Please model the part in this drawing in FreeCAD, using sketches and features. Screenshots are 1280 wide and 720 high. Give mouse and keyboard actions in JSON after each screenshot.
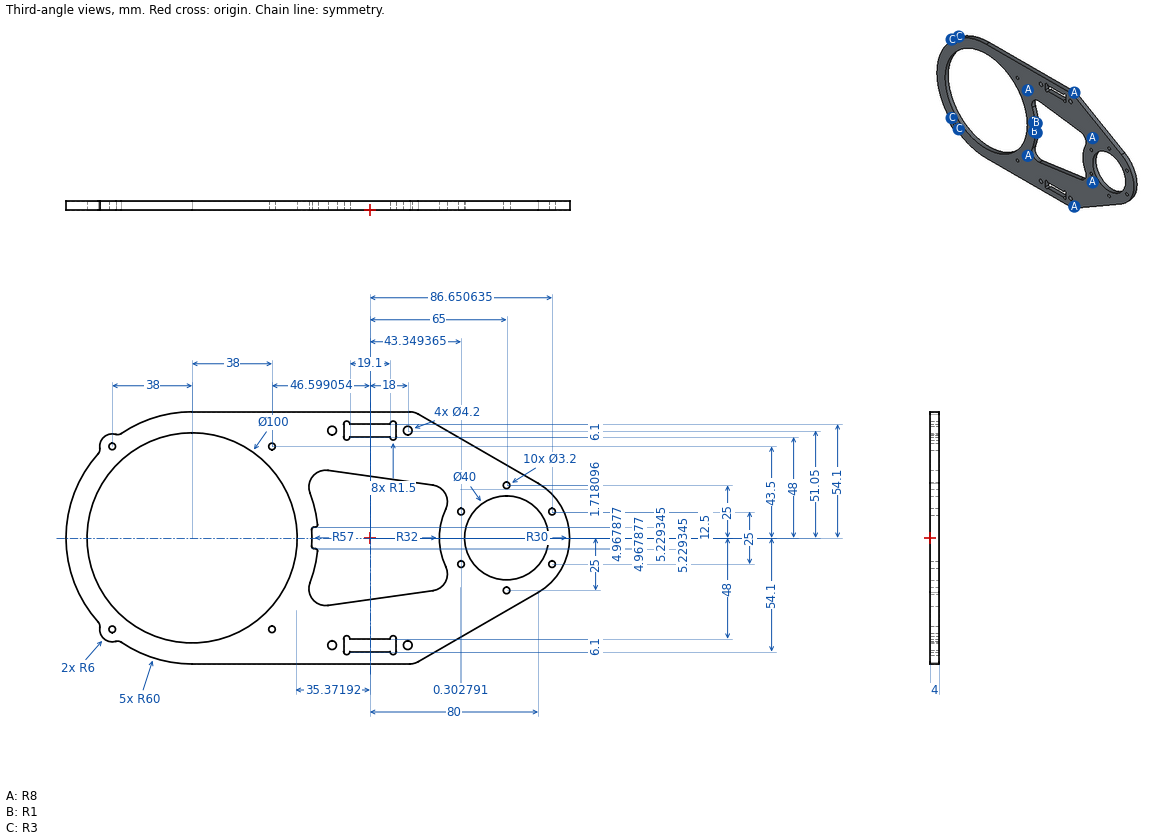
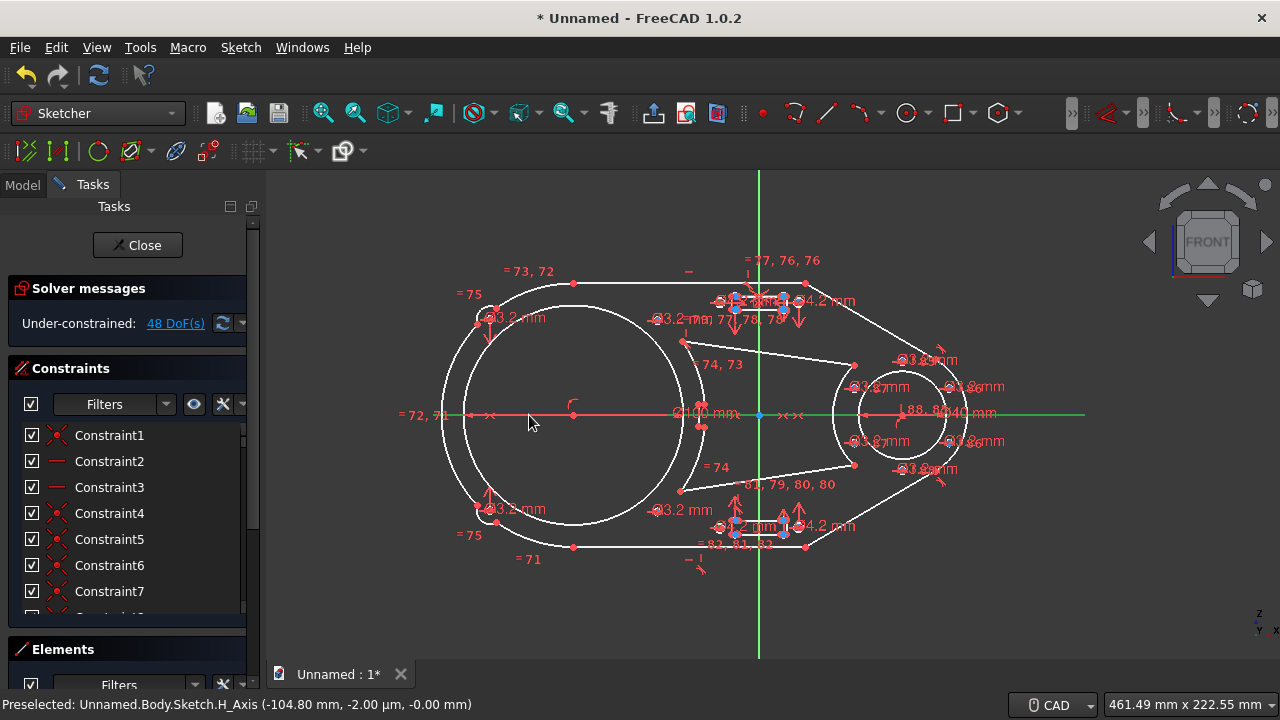
{"action": "key", "text": "s"}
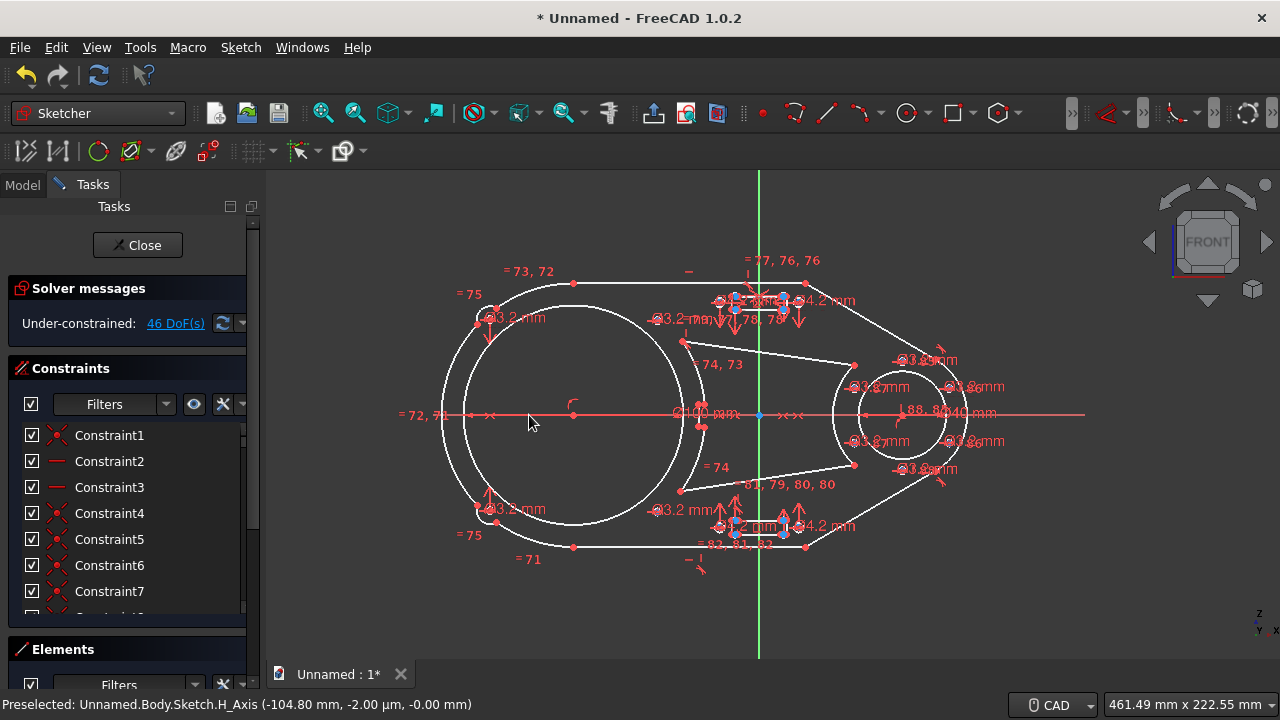
{"action": "left_click", "coordinate": [657, 321]}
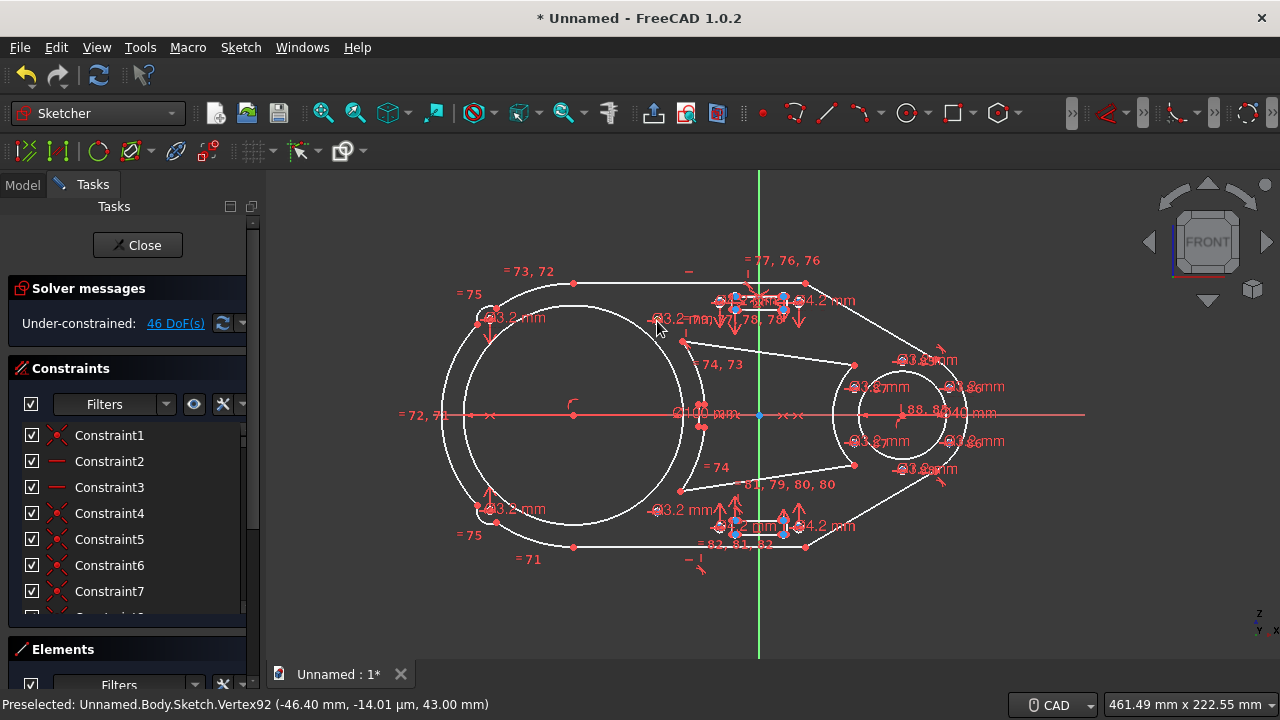
{"action": "left_click", "coordinate": [657, 512]}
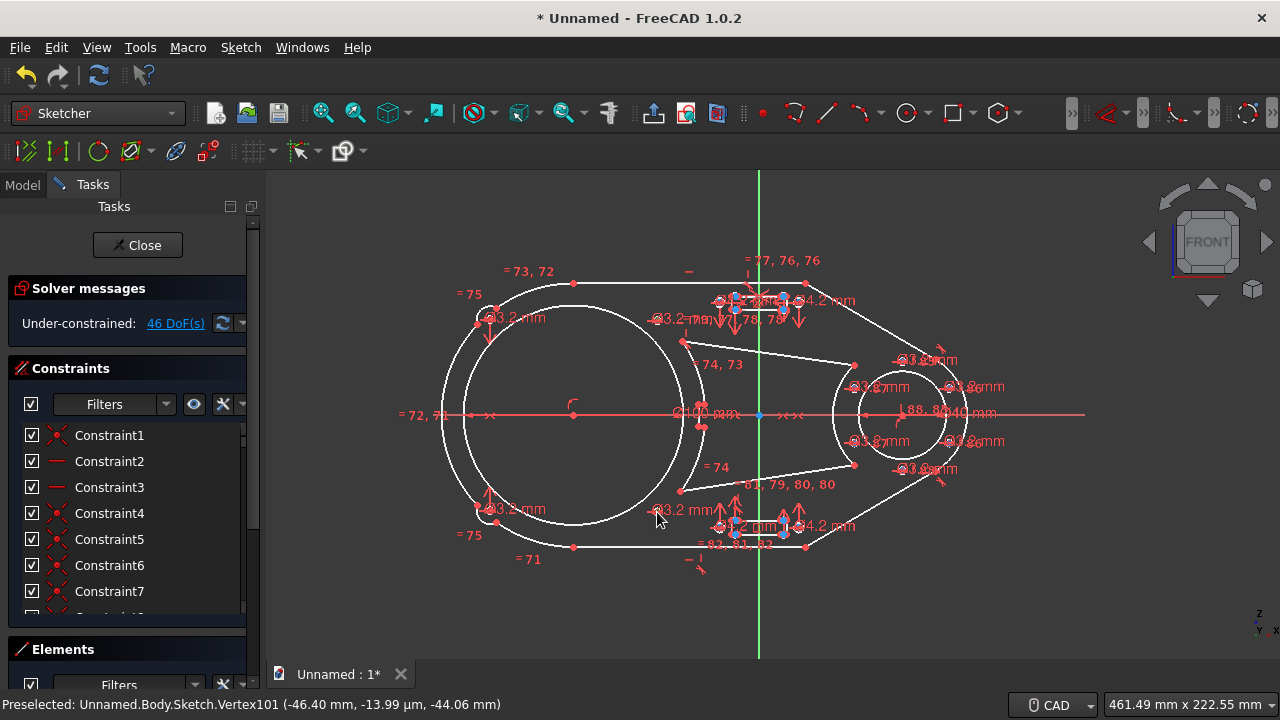
{"action": "left_click", "coordinate": [529, 415]}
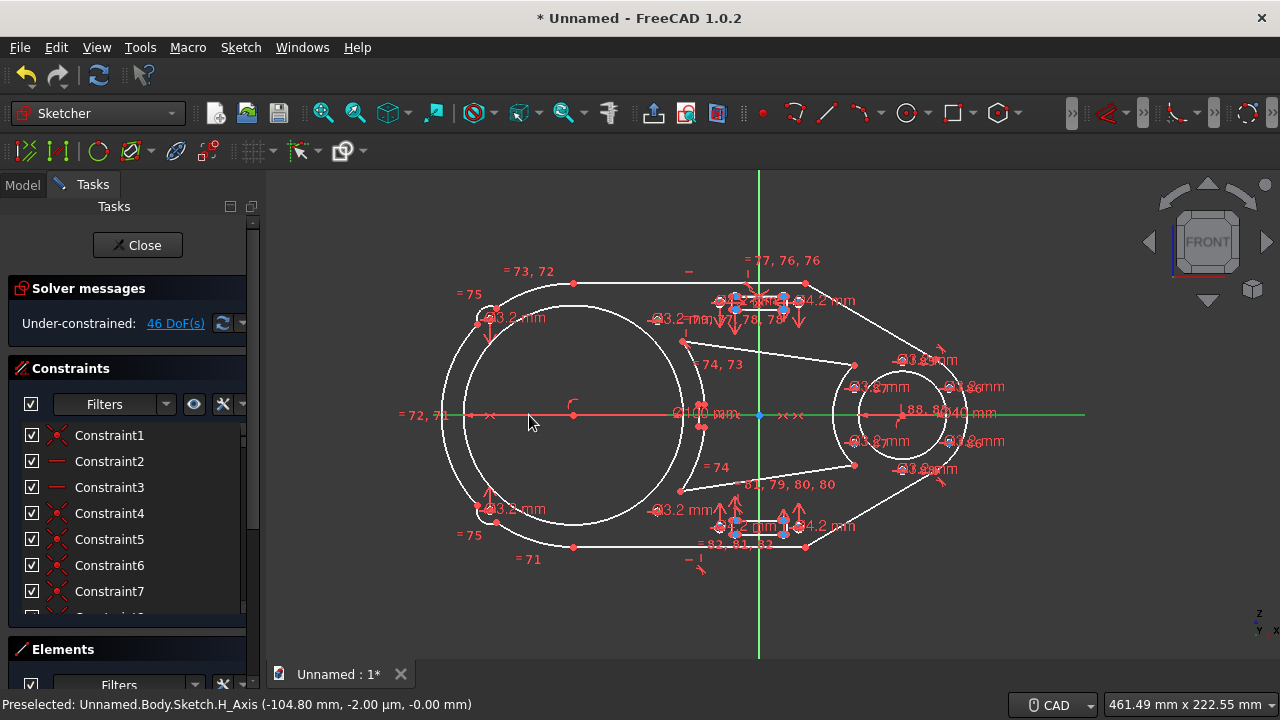
{"action": "key", "text": "s"}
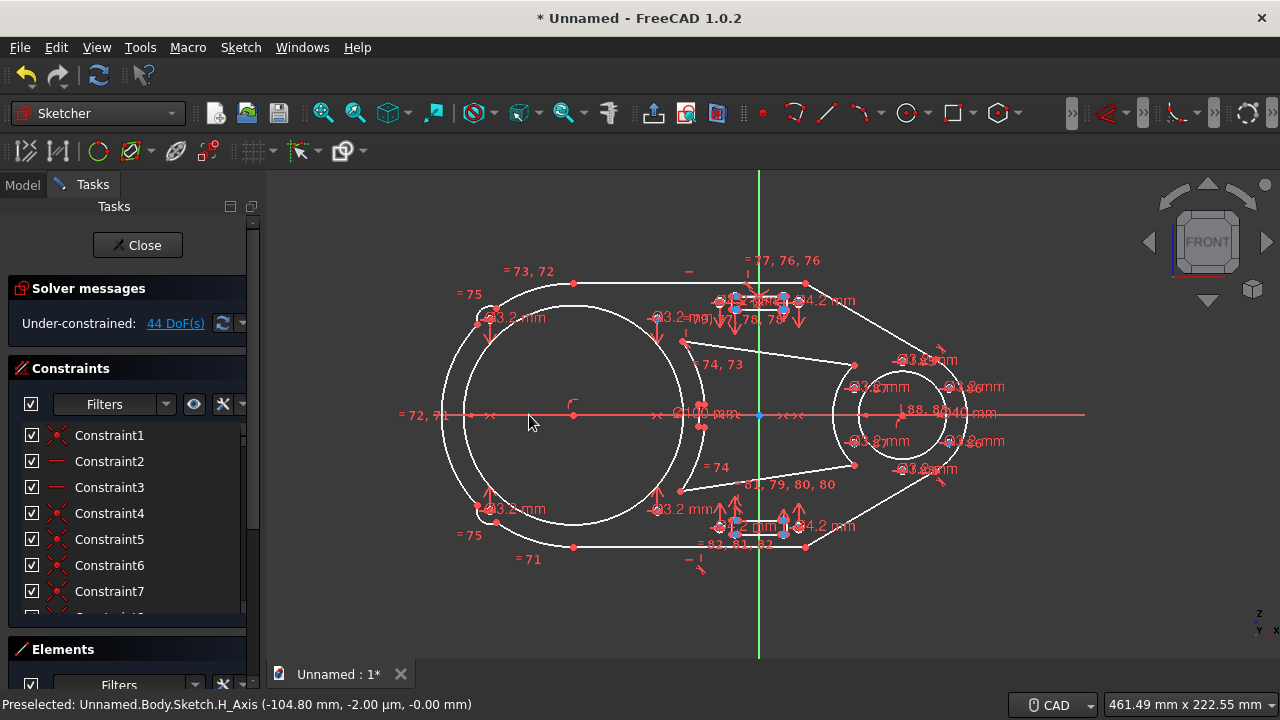
{"action": "left_click", "coordinate": [518, 535]}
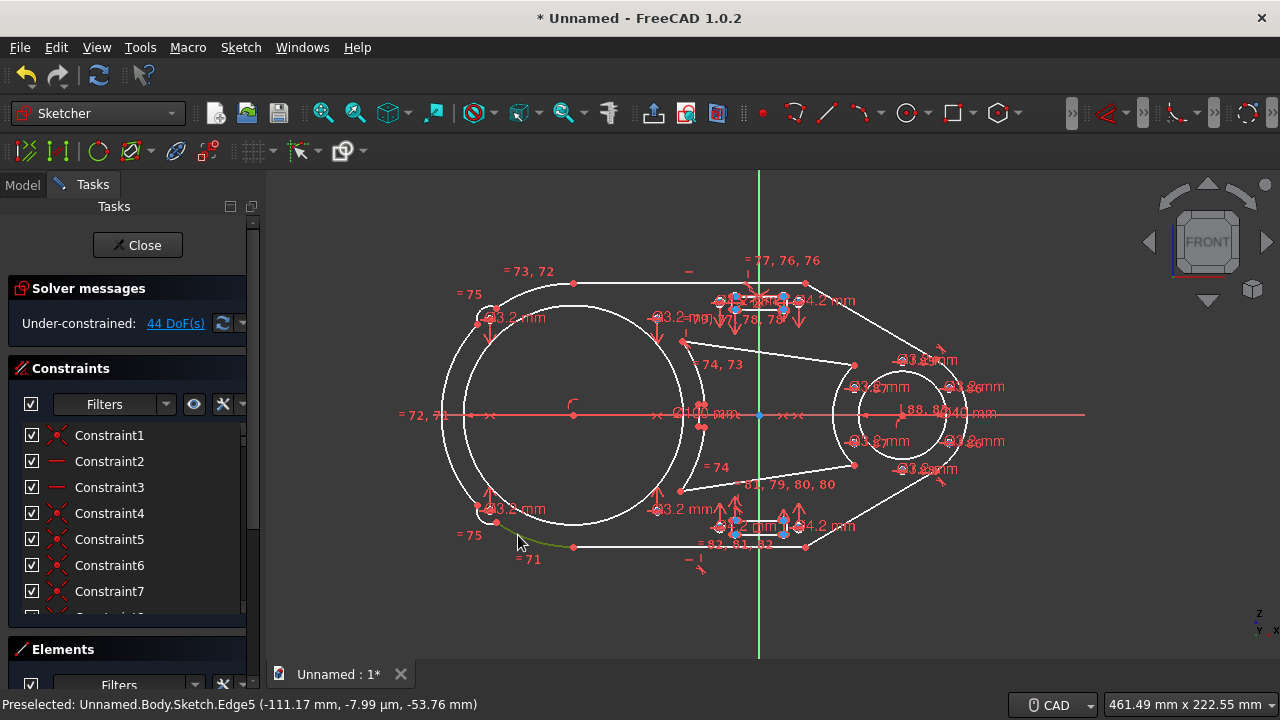
{"action": "key", "text": "k r"}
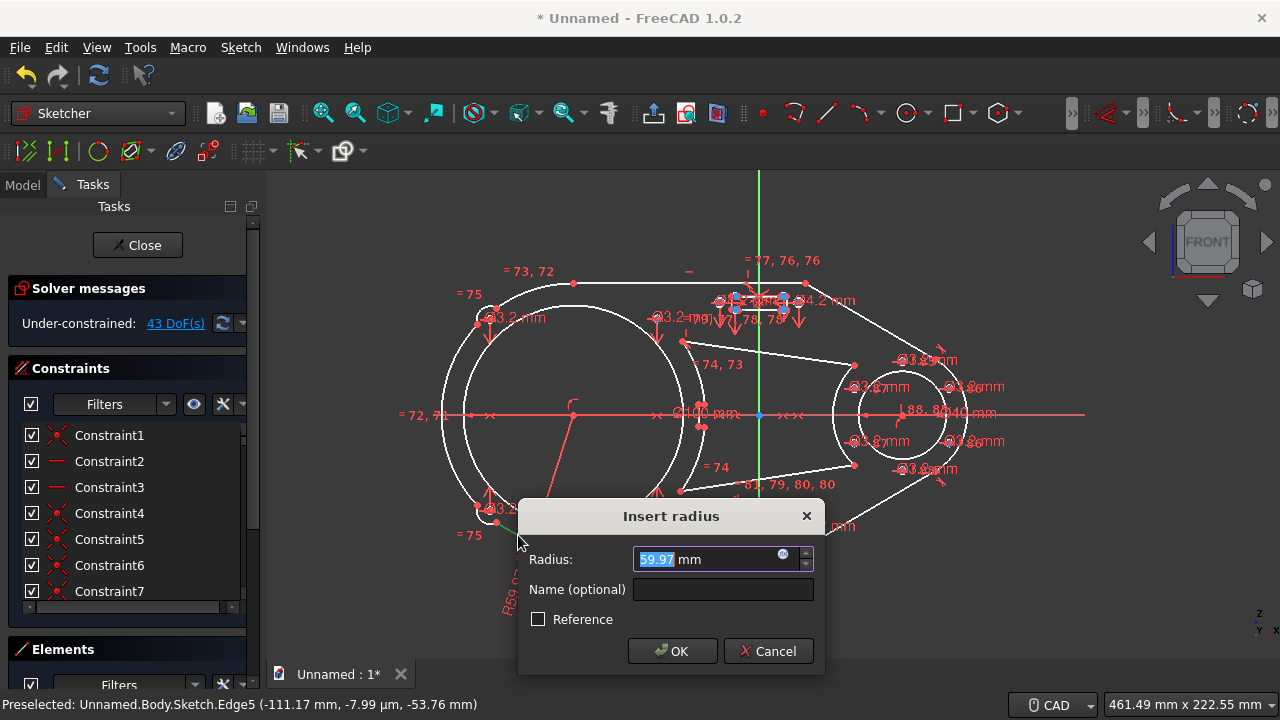
{"action": "type", "text": "60"}
{"action": "key", "text": "Return"}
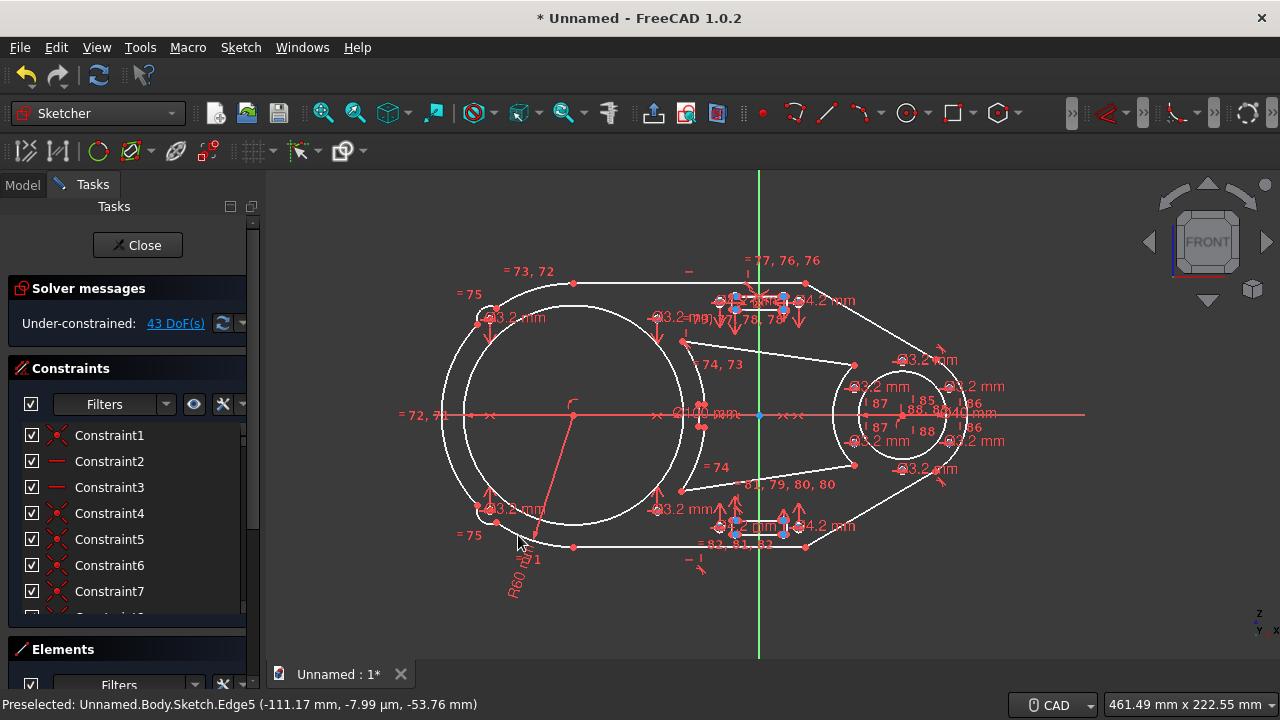
{"action": "scroll", "coordinate": [478, 516], "scroll_direction": "up", "scroll_amount": 6}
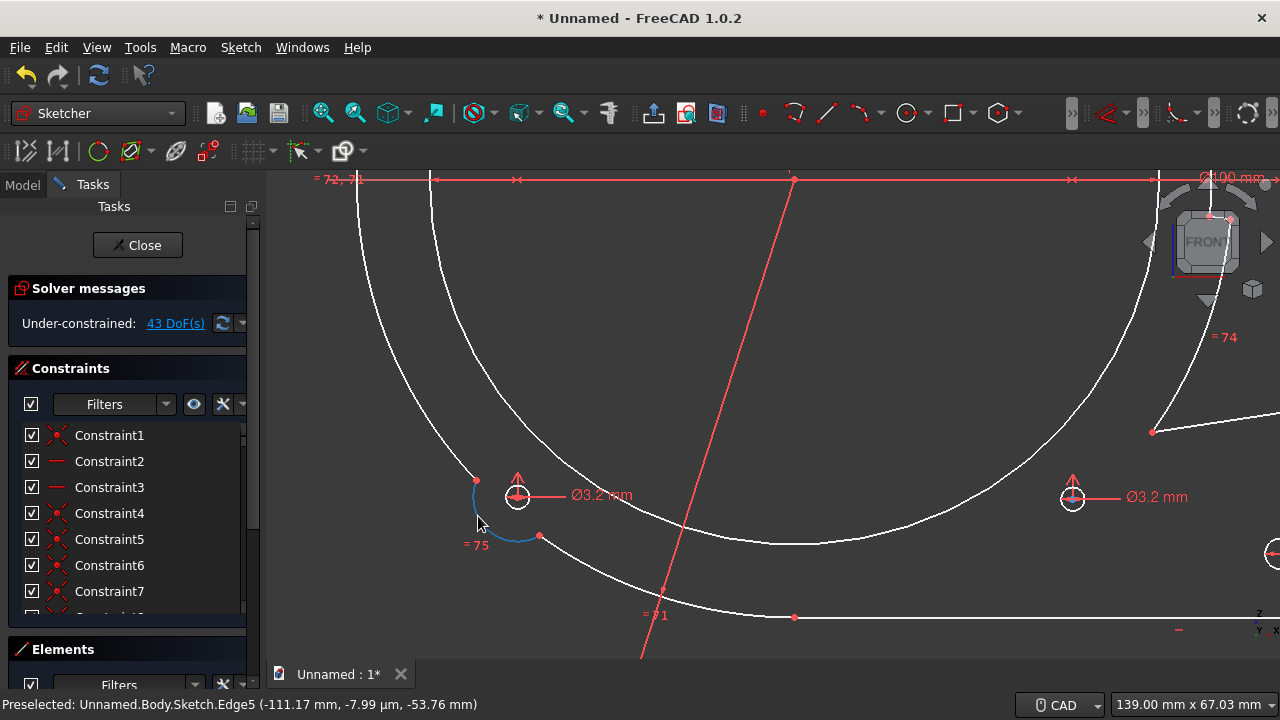
{"action": "left_click", "coordinate": [476, 513]}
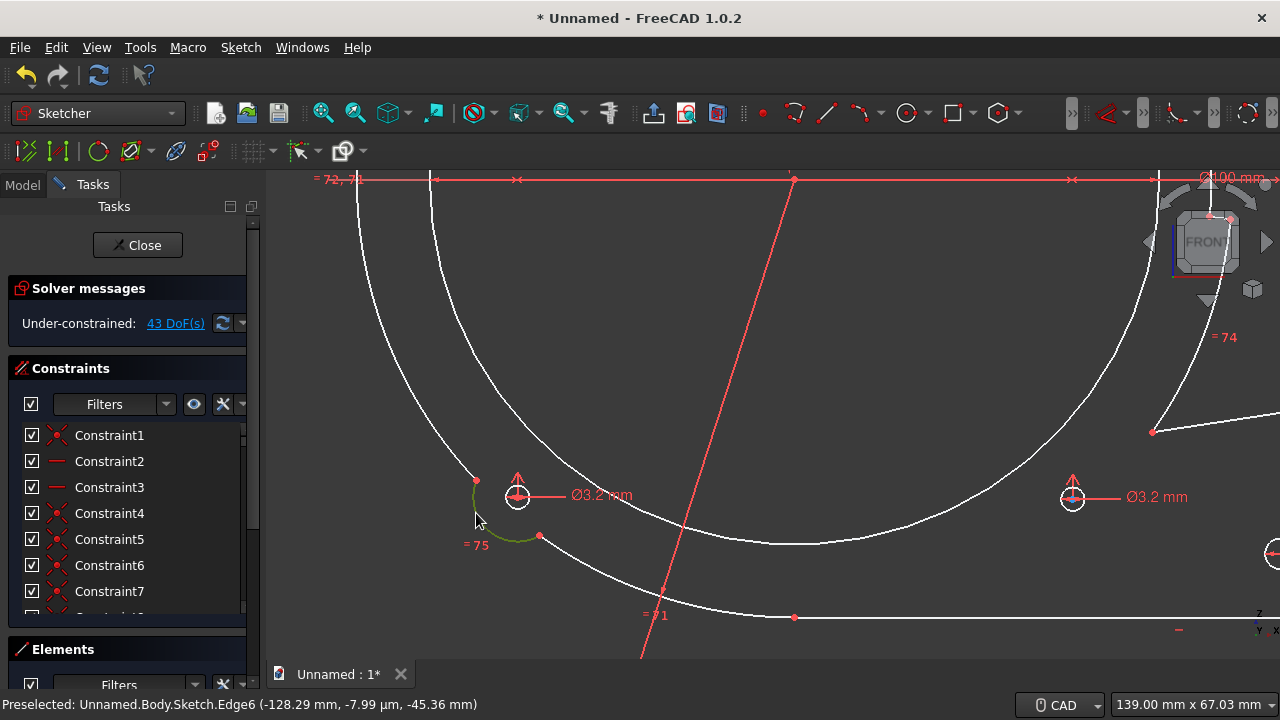
{"action": "left_click", "coordinate": [1128, 114]}